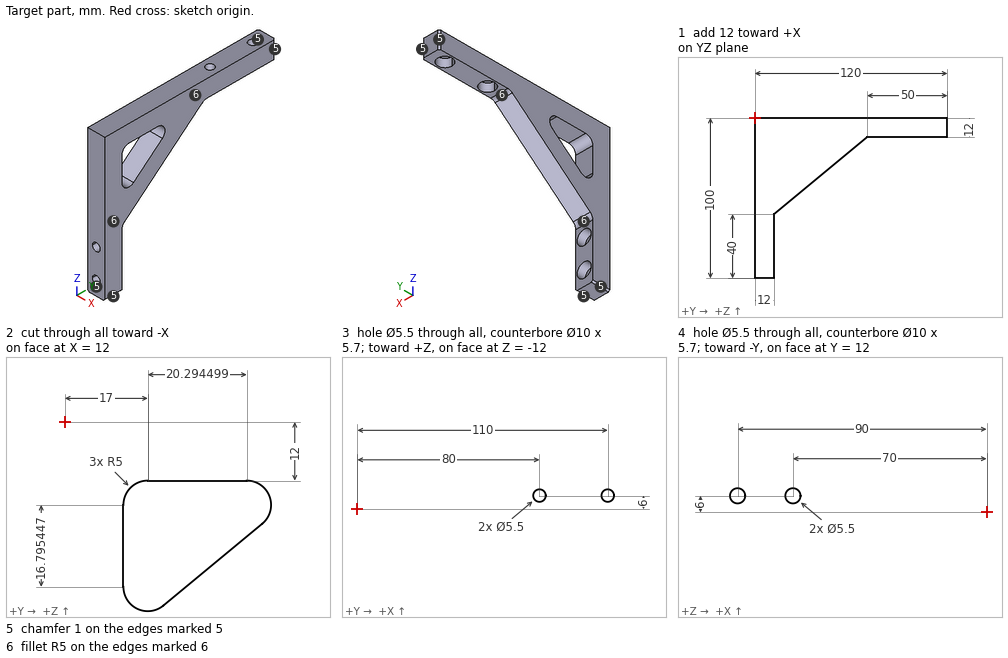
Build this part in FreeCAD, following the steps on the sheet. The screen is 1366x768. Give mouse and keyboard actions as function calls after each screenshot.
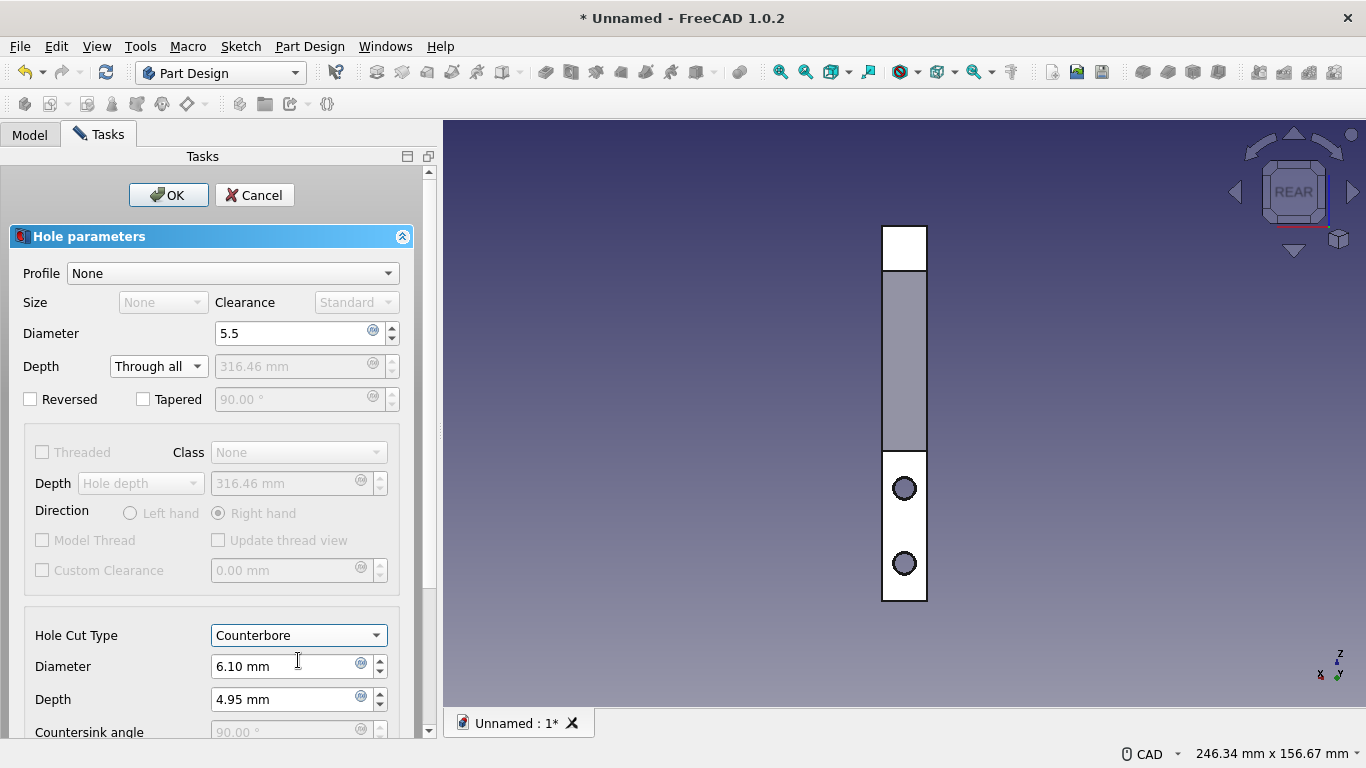
triple_click(292, 666)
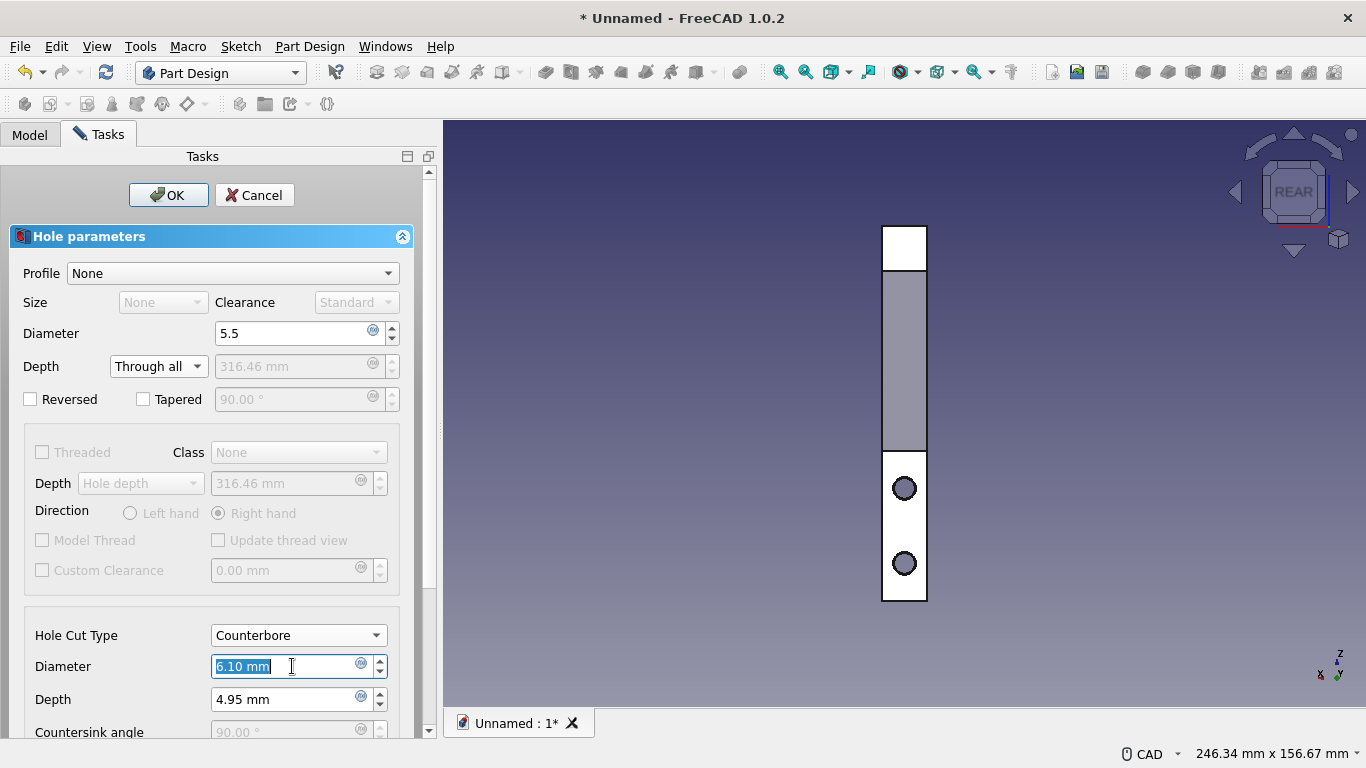
text(10)
key(Tab)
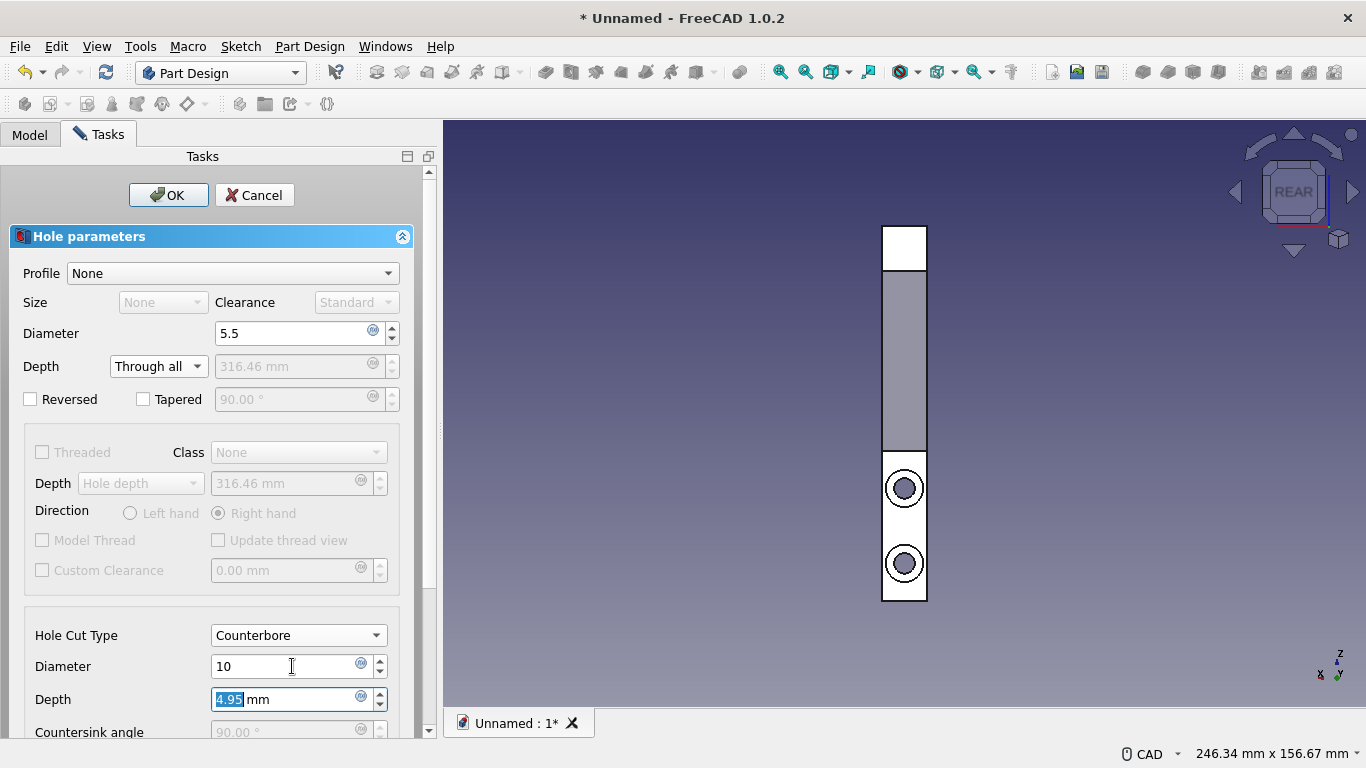
text(5.7)
key(Tab)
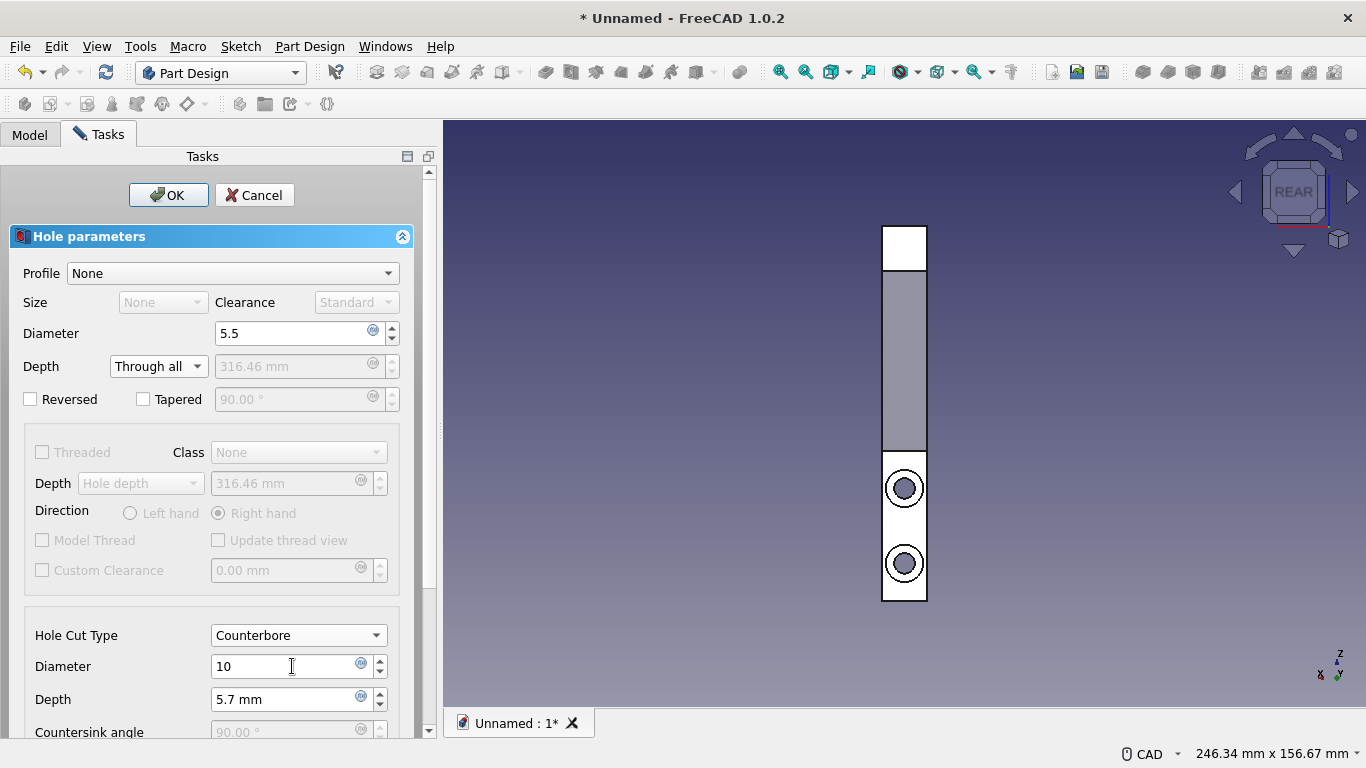
click(169, 195)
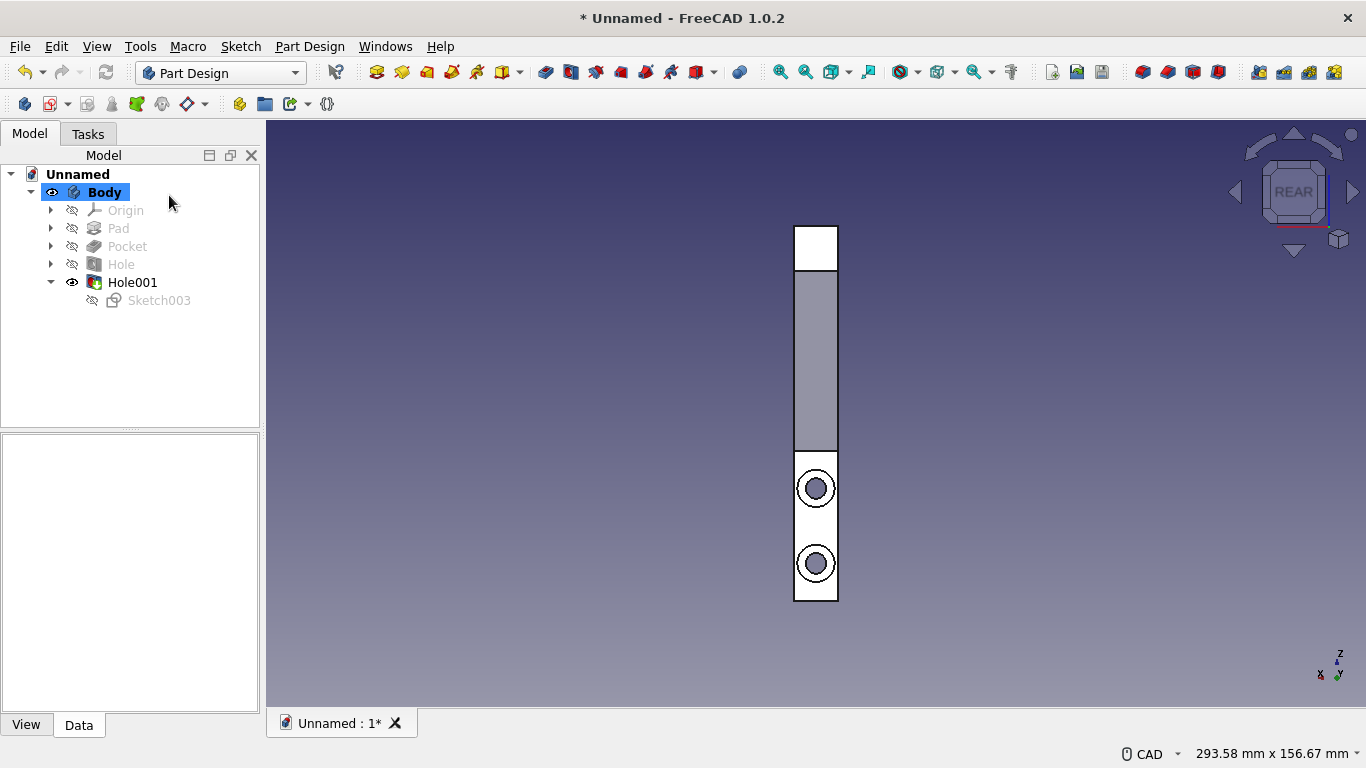
click(838, 248)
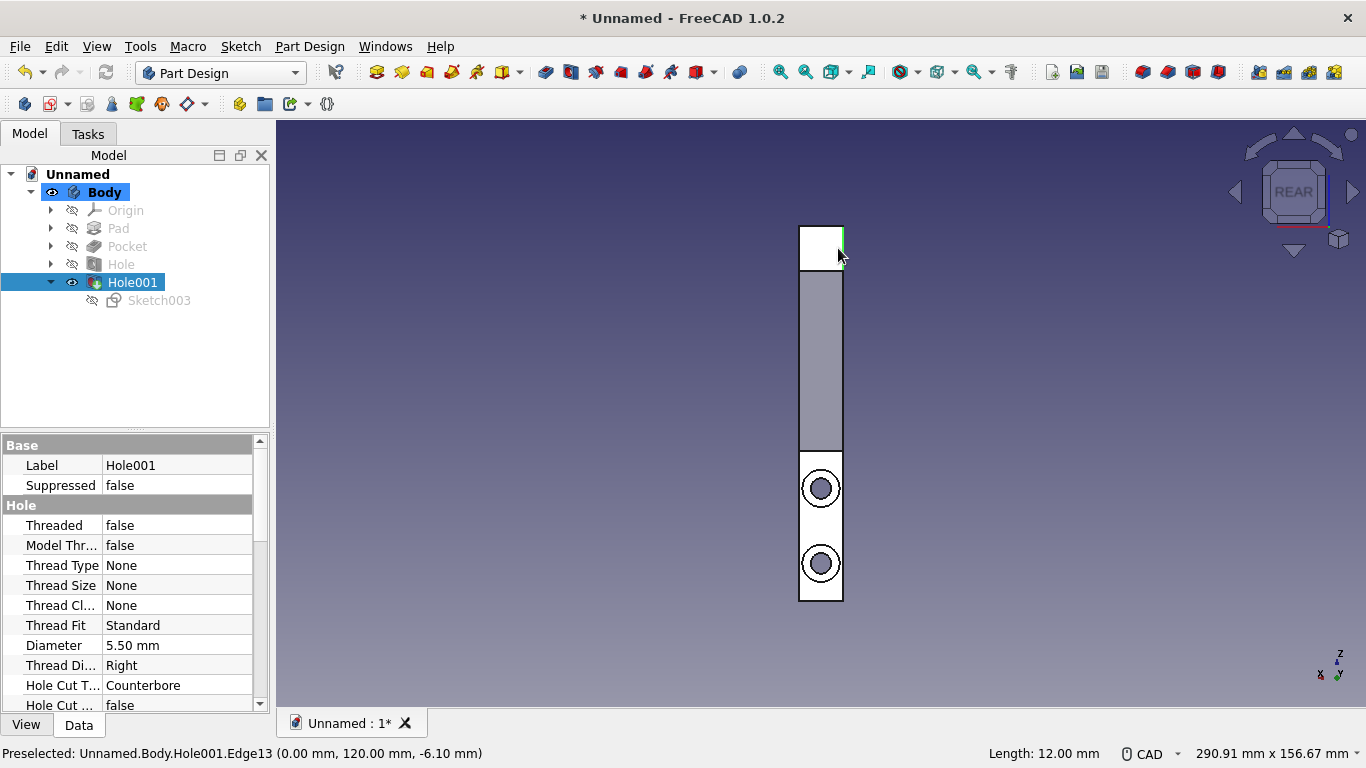
key(0)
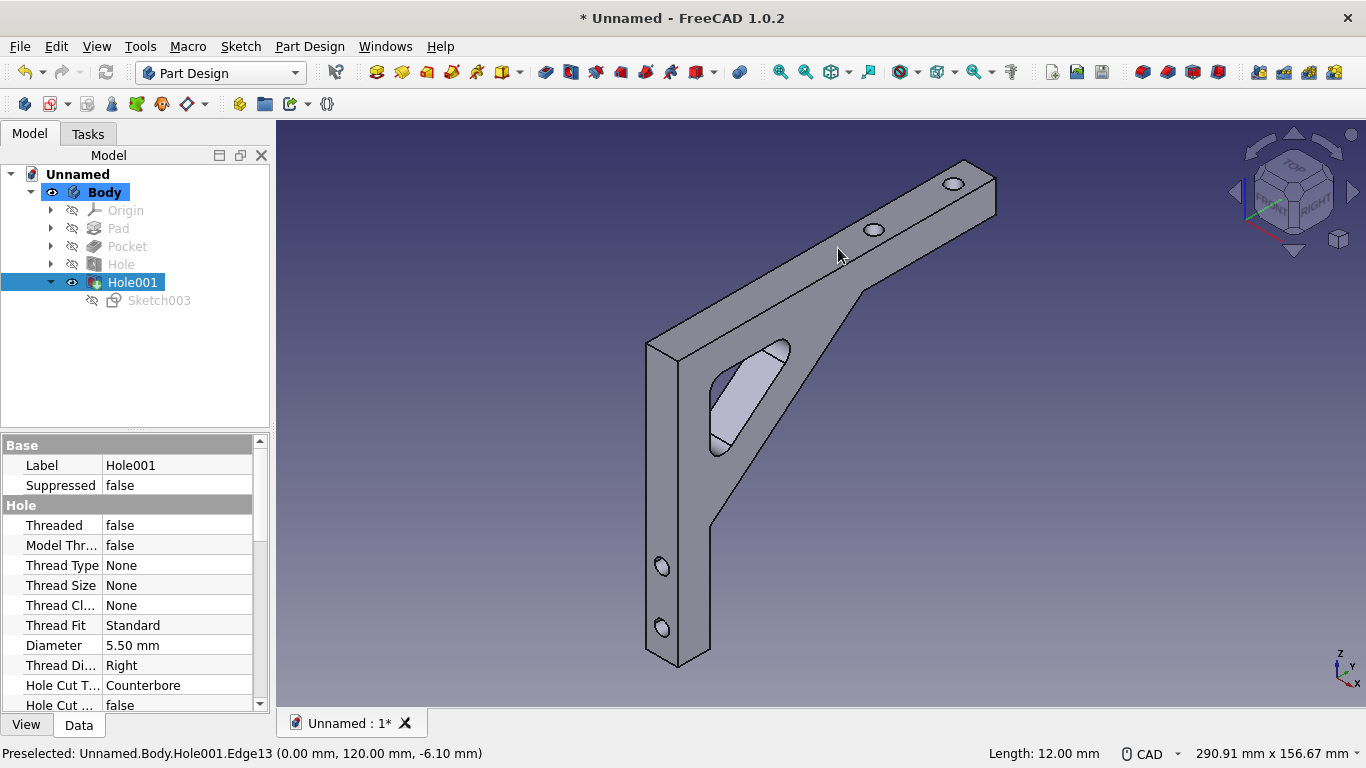
key(2)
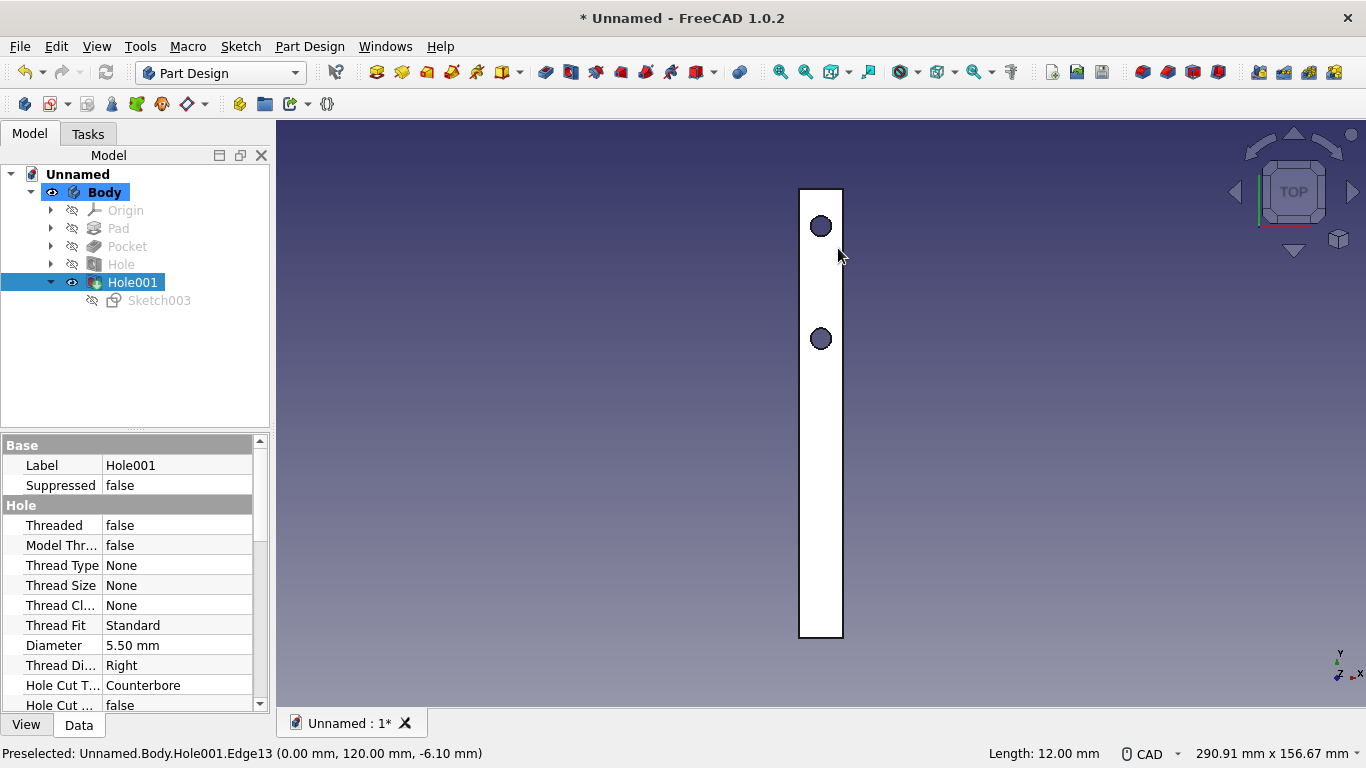
key(1)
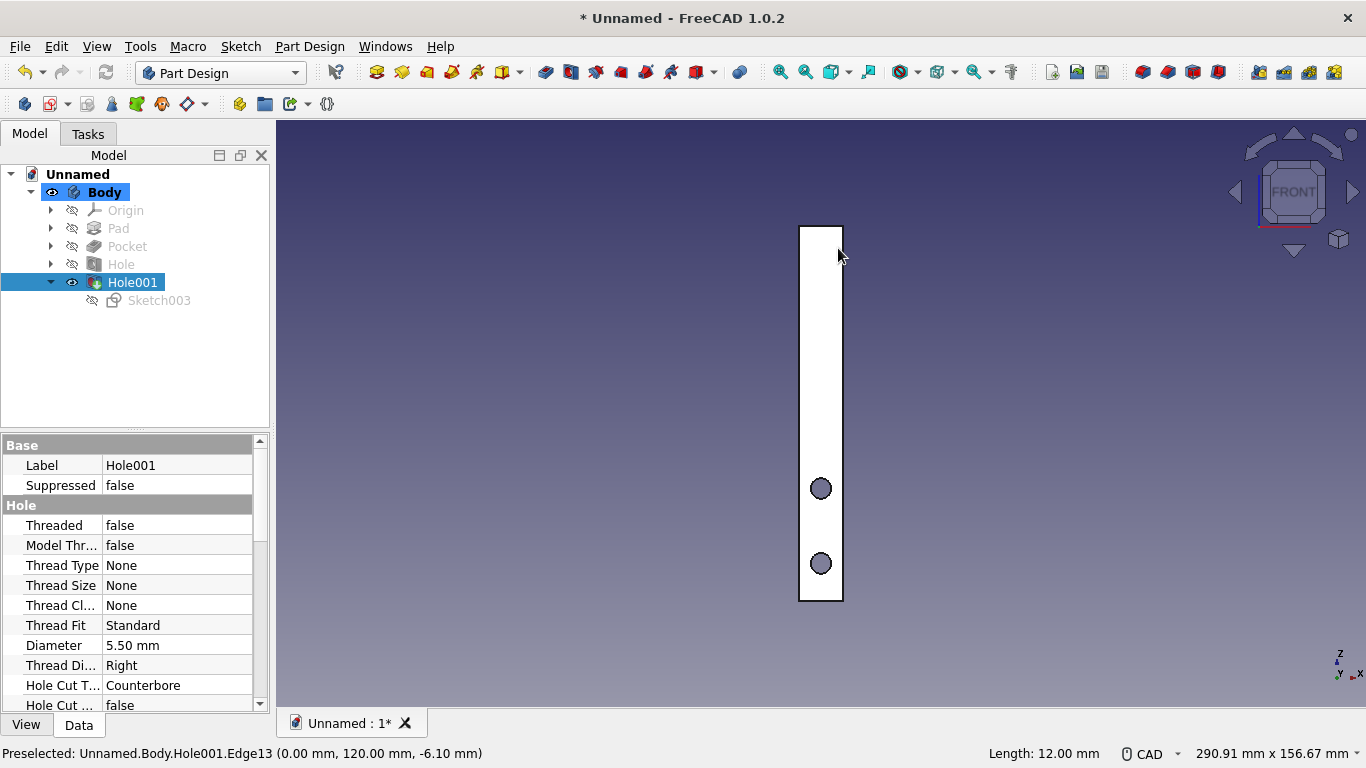
key(3)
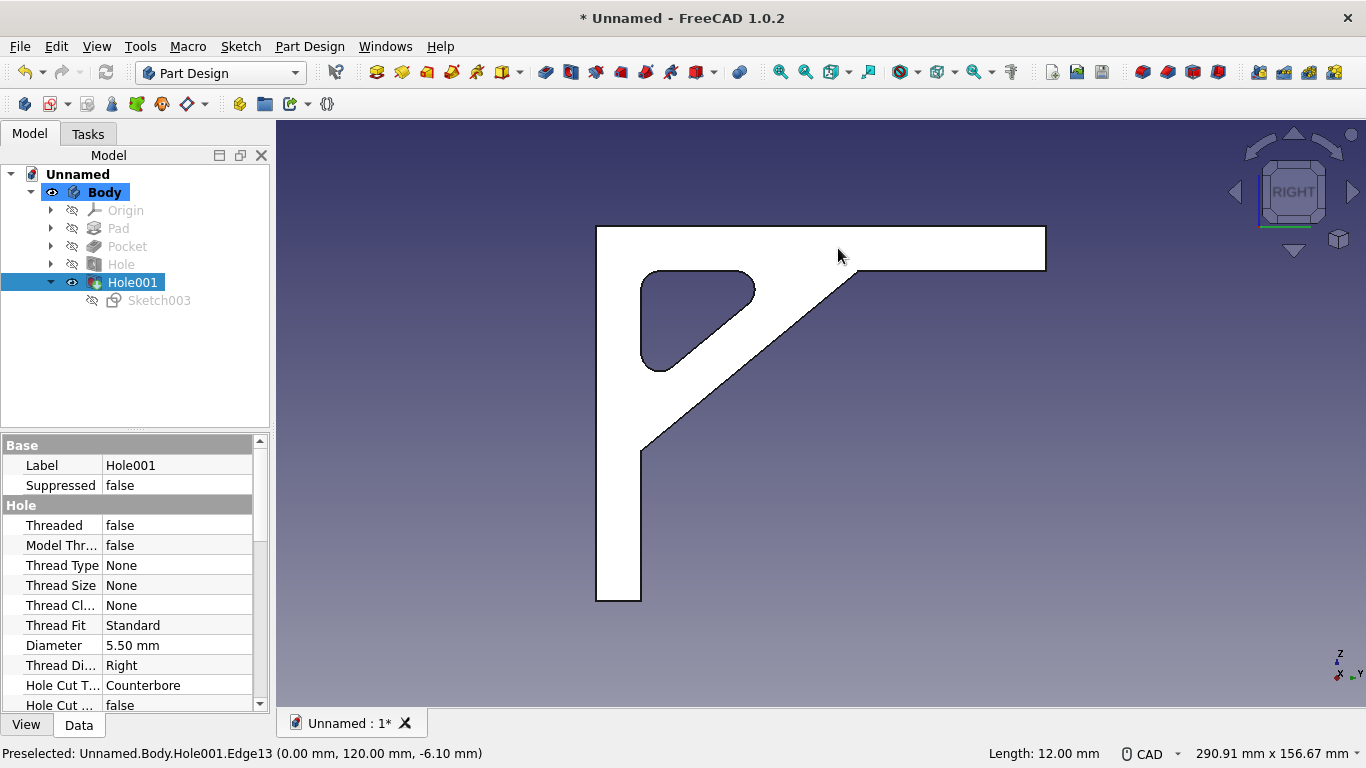
click(1046, 248, ctrl)